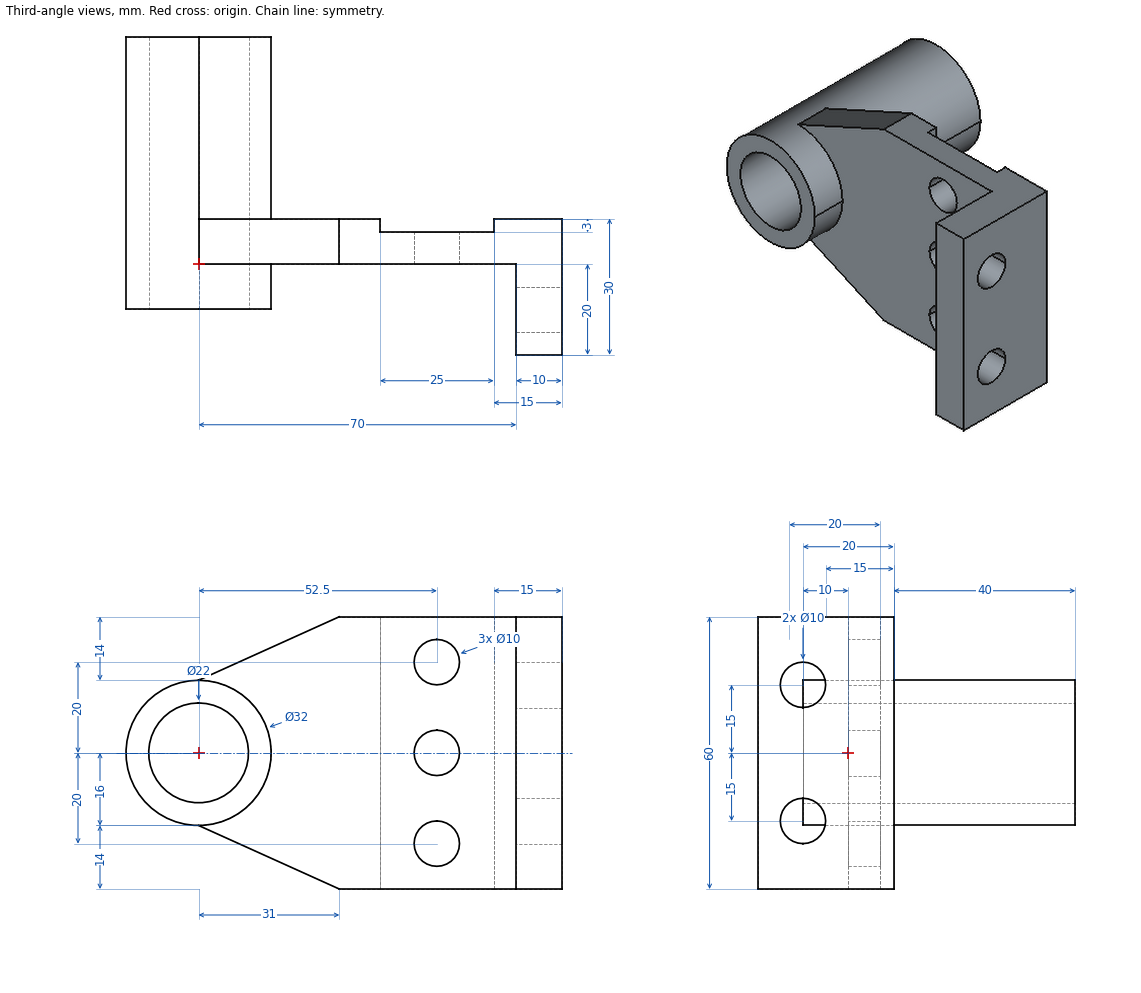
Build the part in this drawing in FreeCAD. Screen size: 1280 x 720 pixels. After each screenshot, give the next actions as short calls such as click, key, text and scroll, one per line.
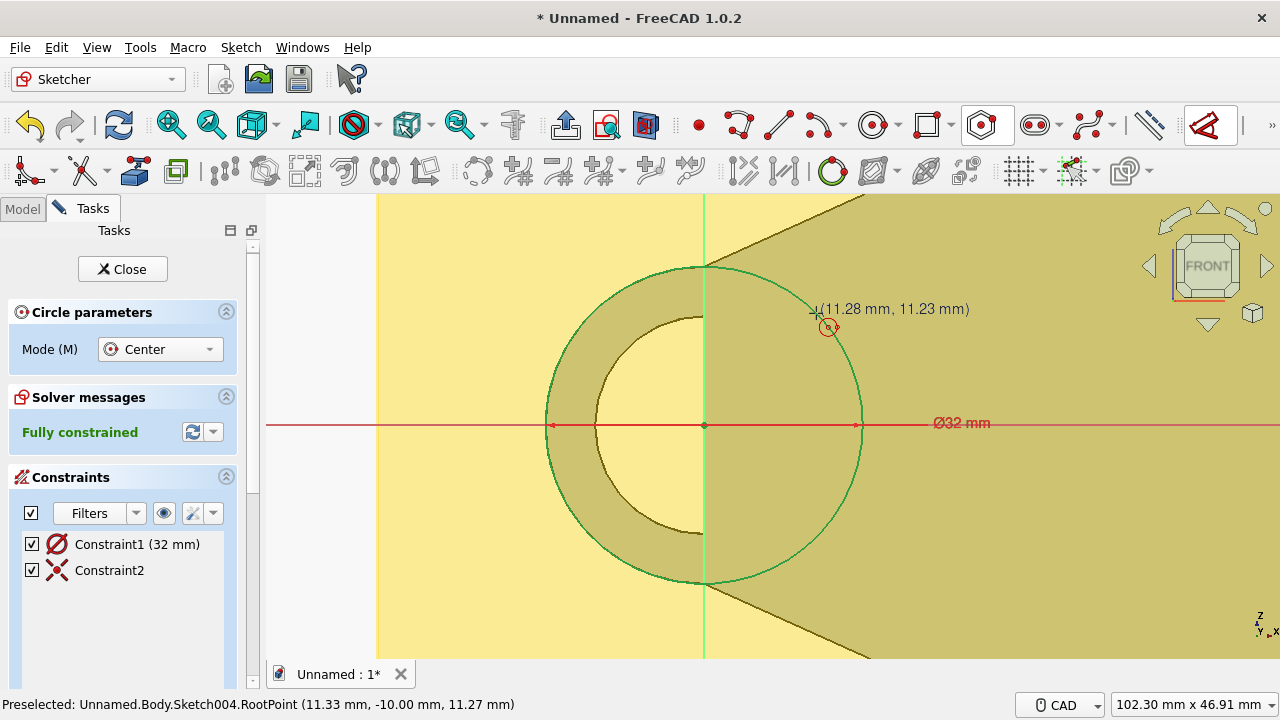
click(704, 425)
move(781, 348)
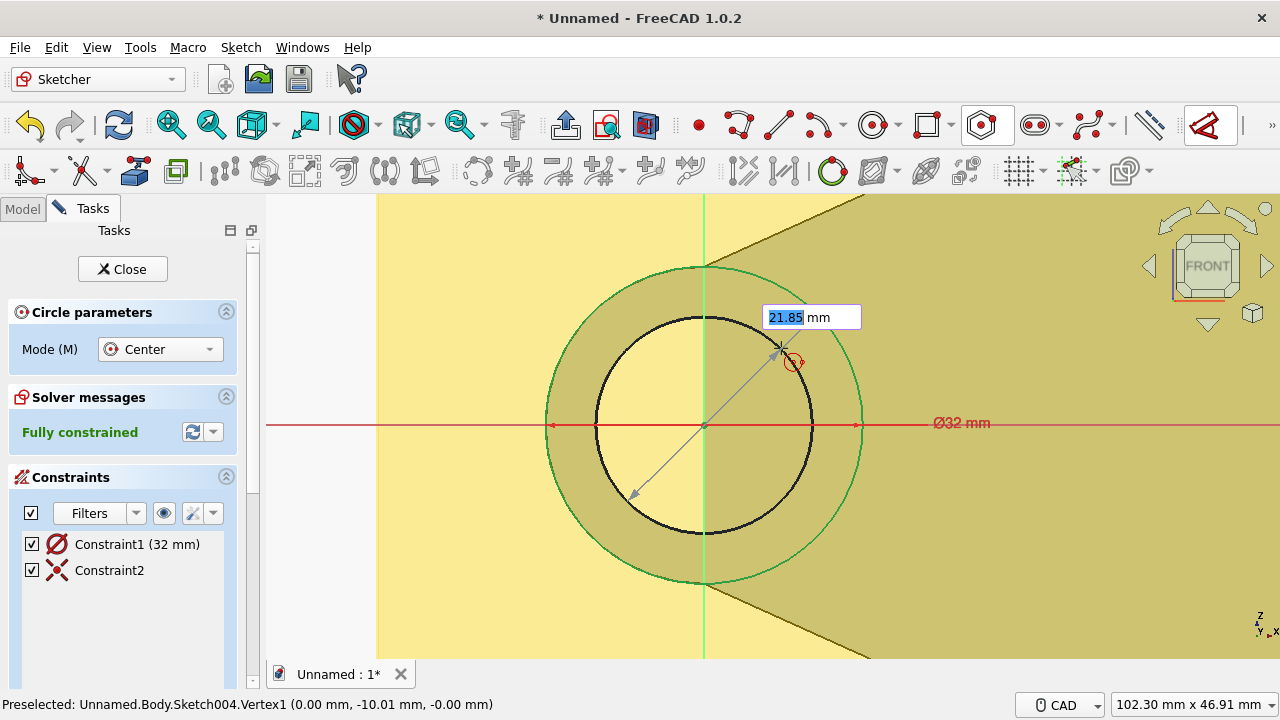
text(22)
key(Return)
key(Escape)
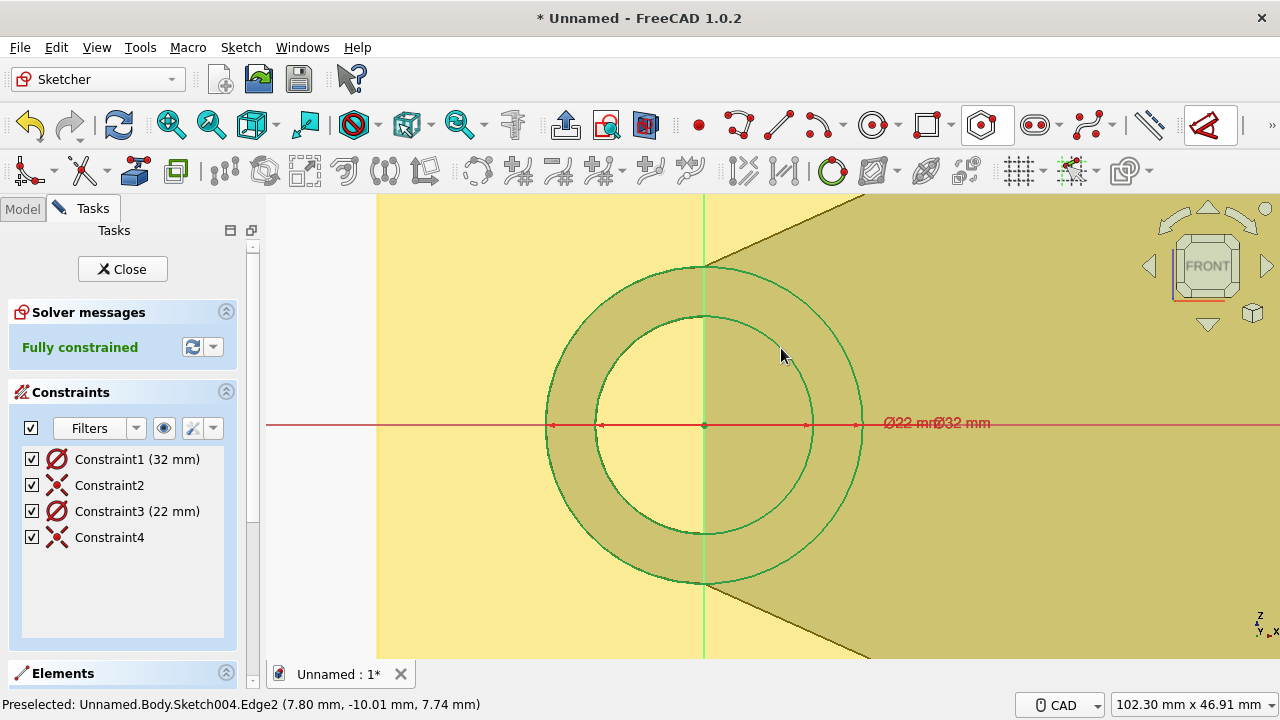
click(123, 269)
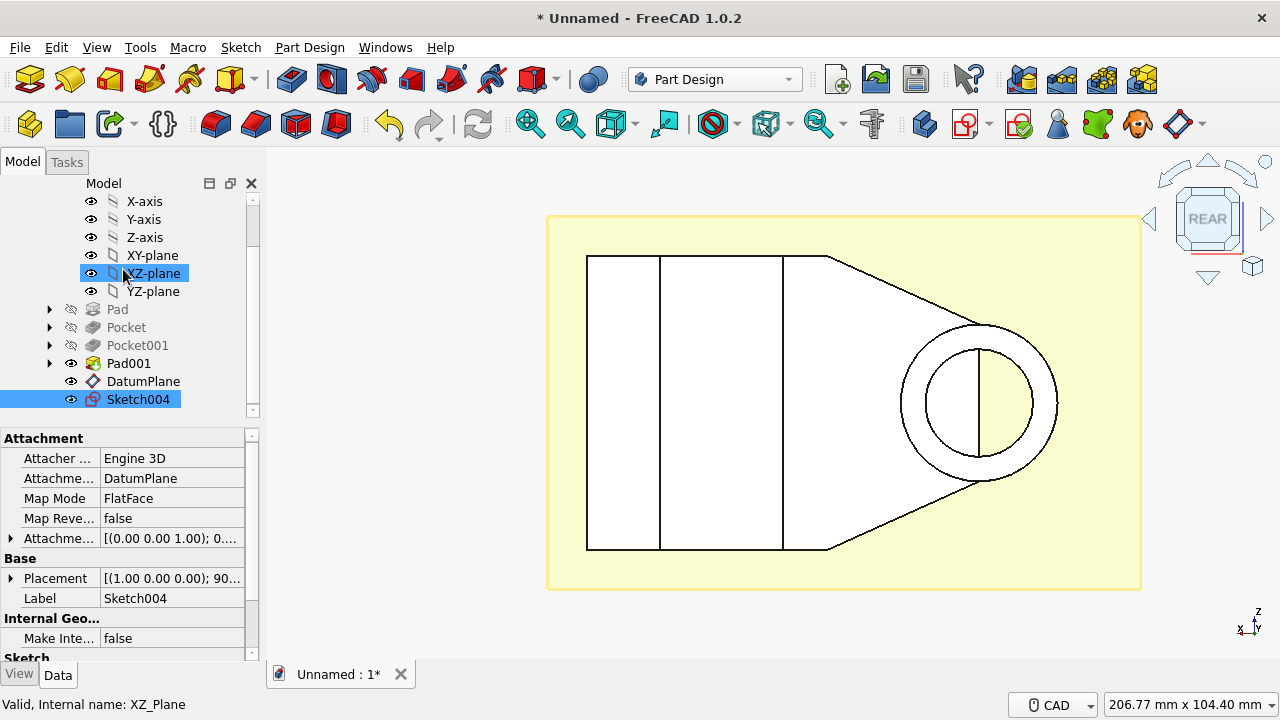
click(30, 80)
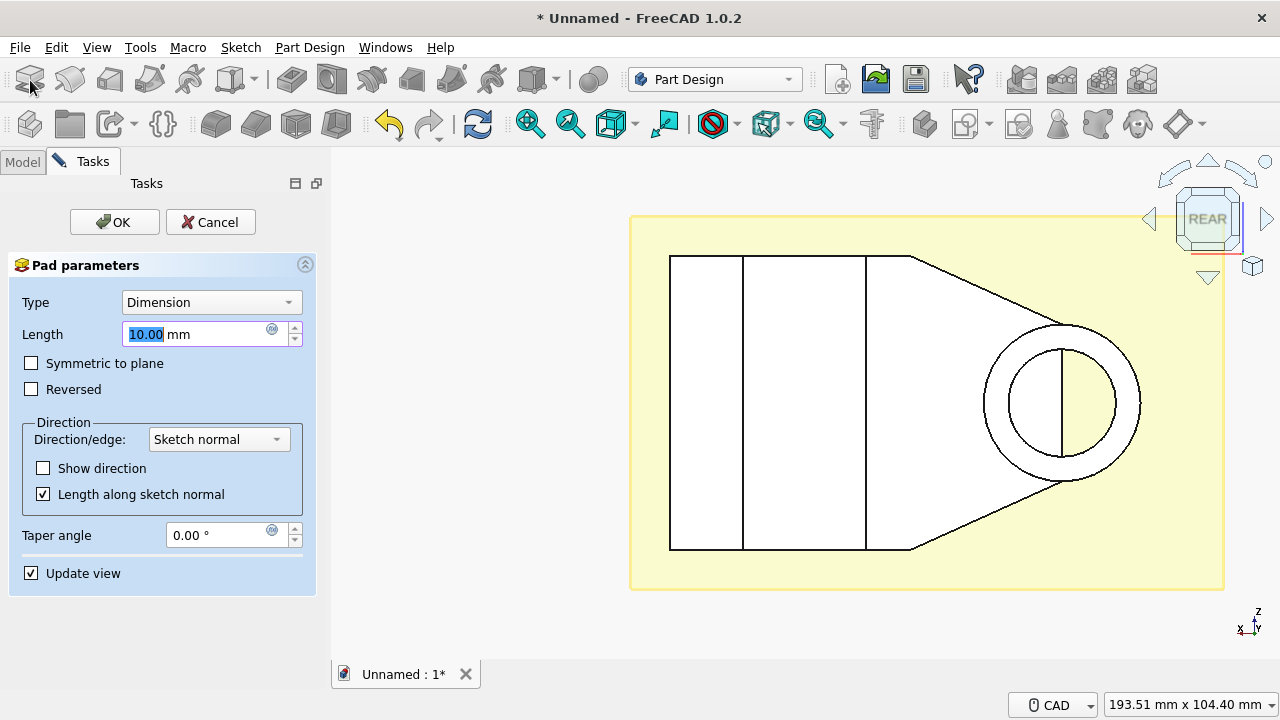
text(20)
key(Tab)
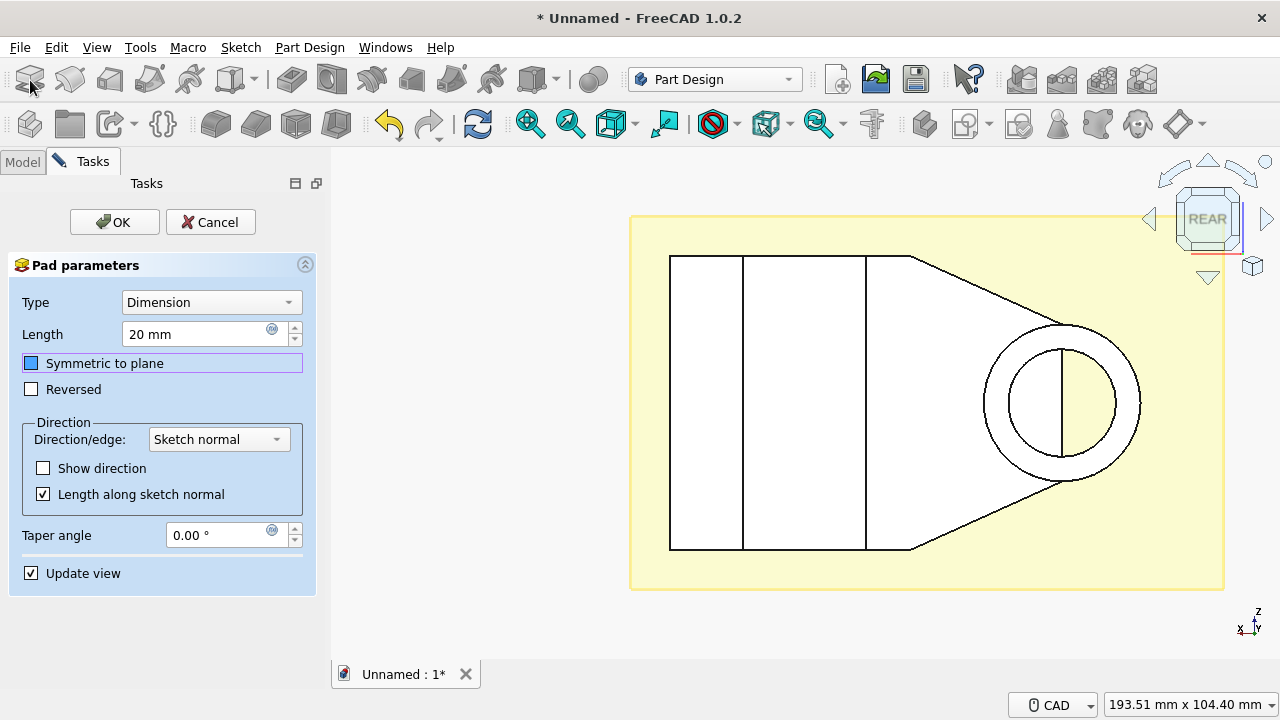
click(30, 389)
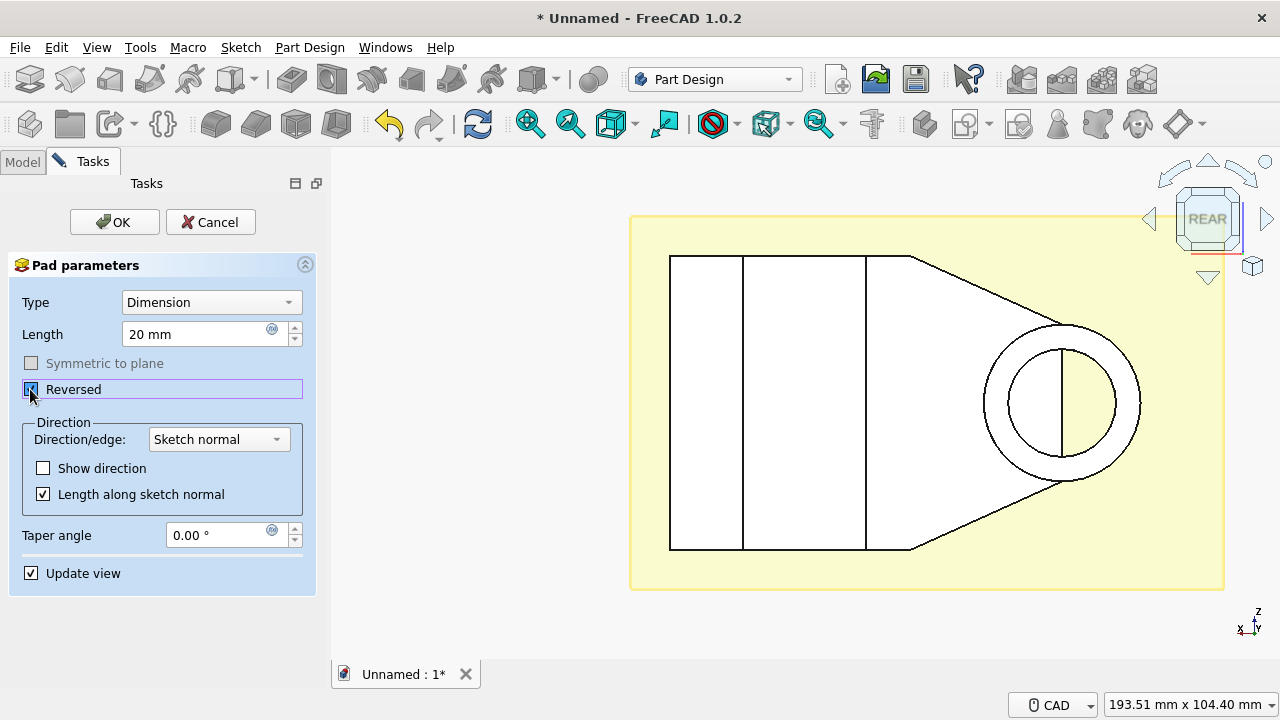
click(115, 222)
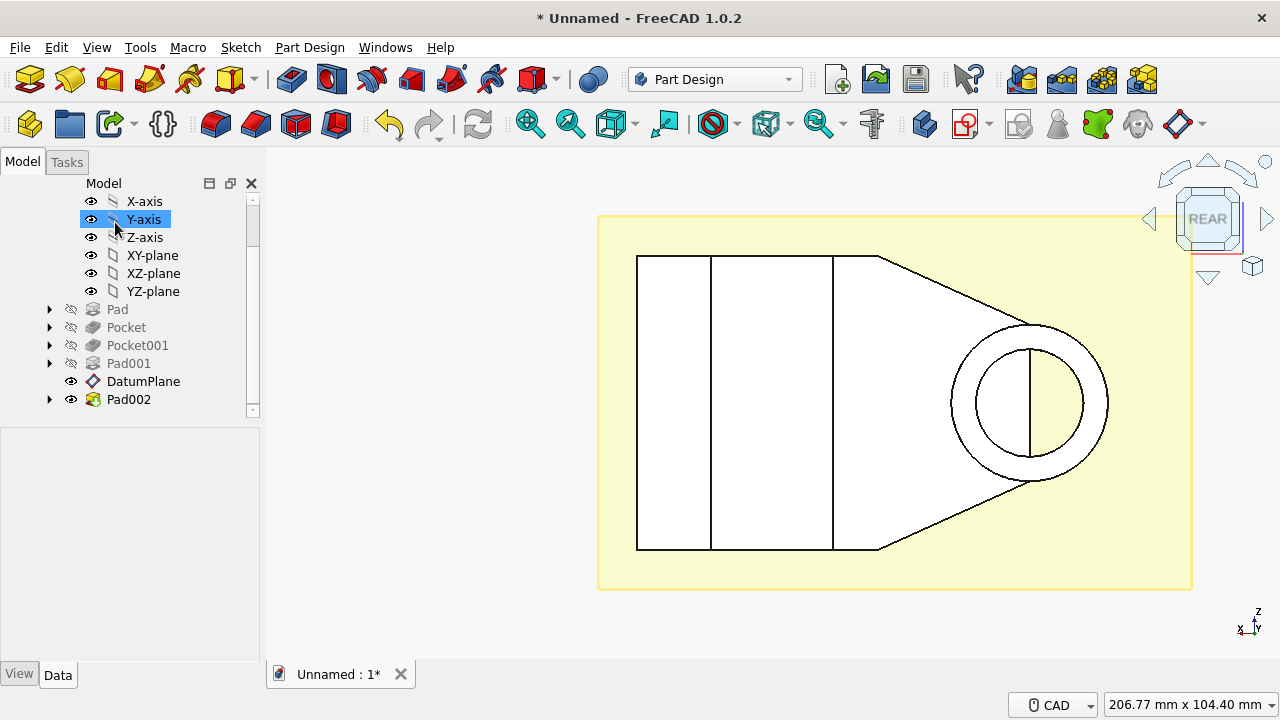
click(116, 381)
key(space)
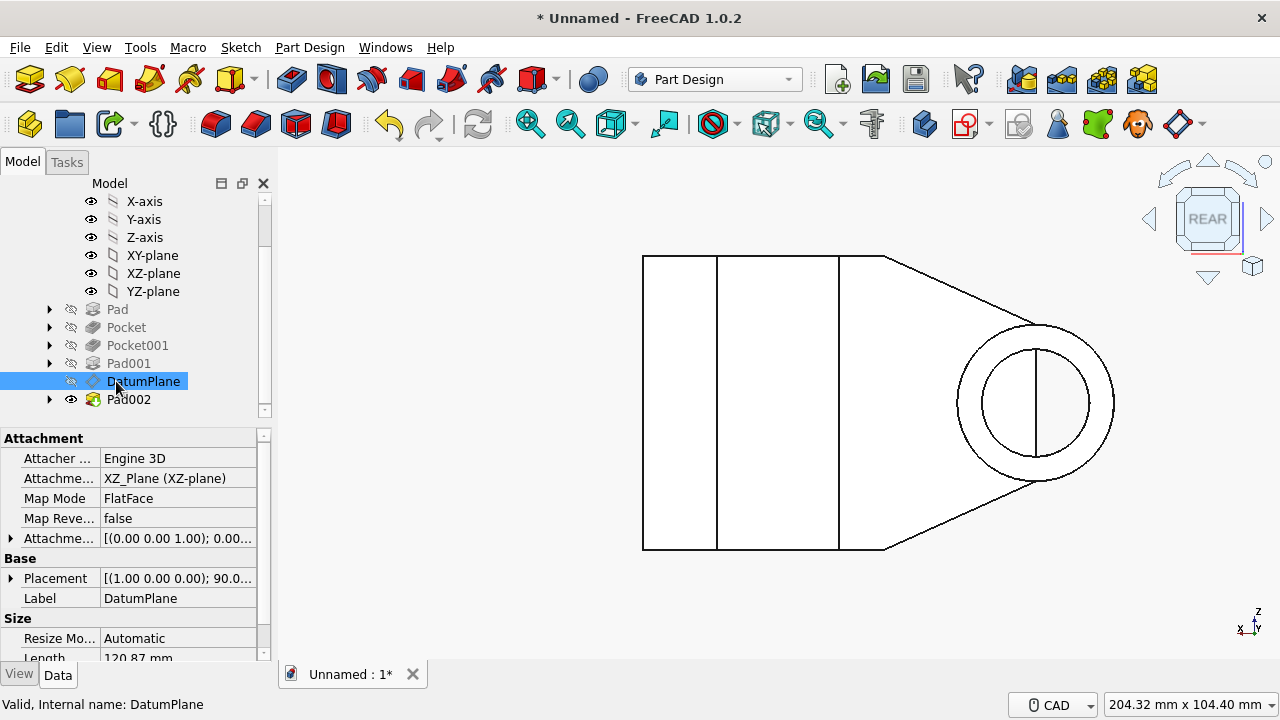
key(0)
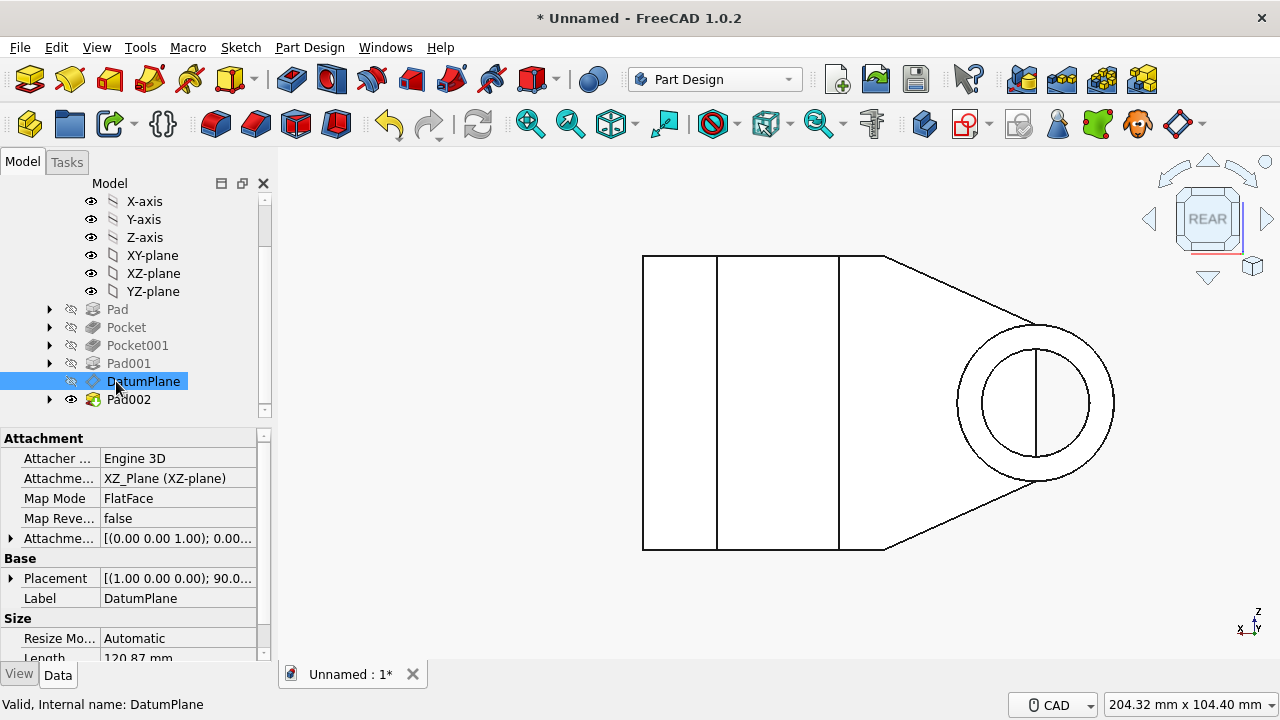
key(v)
key(f)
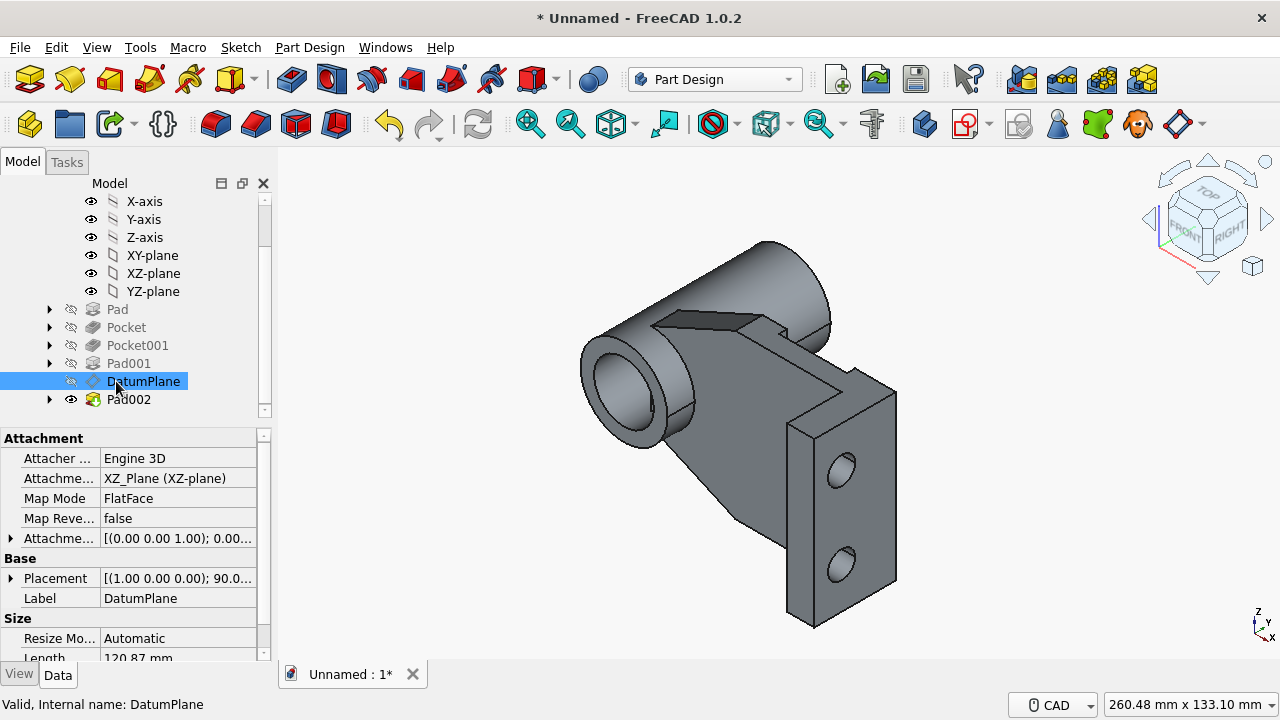
click(599, 348)